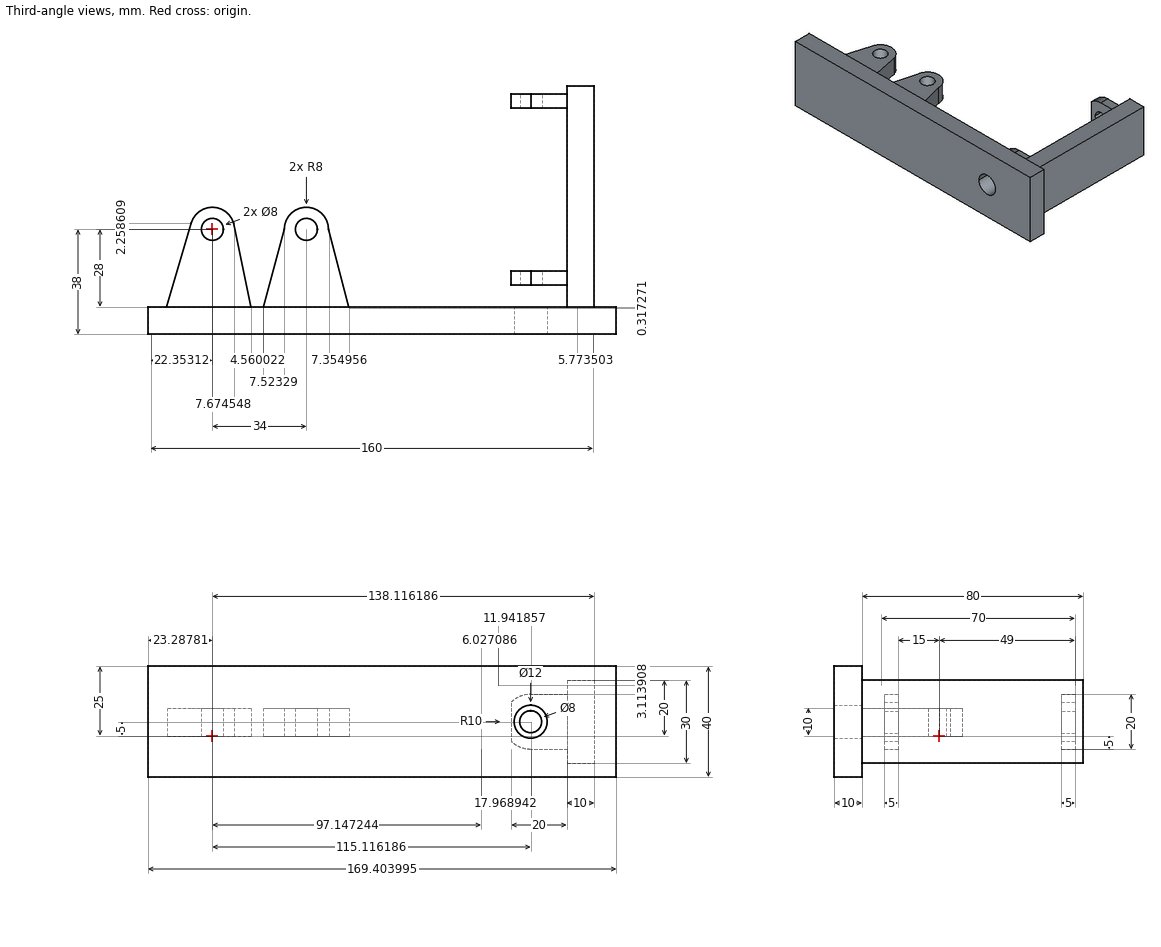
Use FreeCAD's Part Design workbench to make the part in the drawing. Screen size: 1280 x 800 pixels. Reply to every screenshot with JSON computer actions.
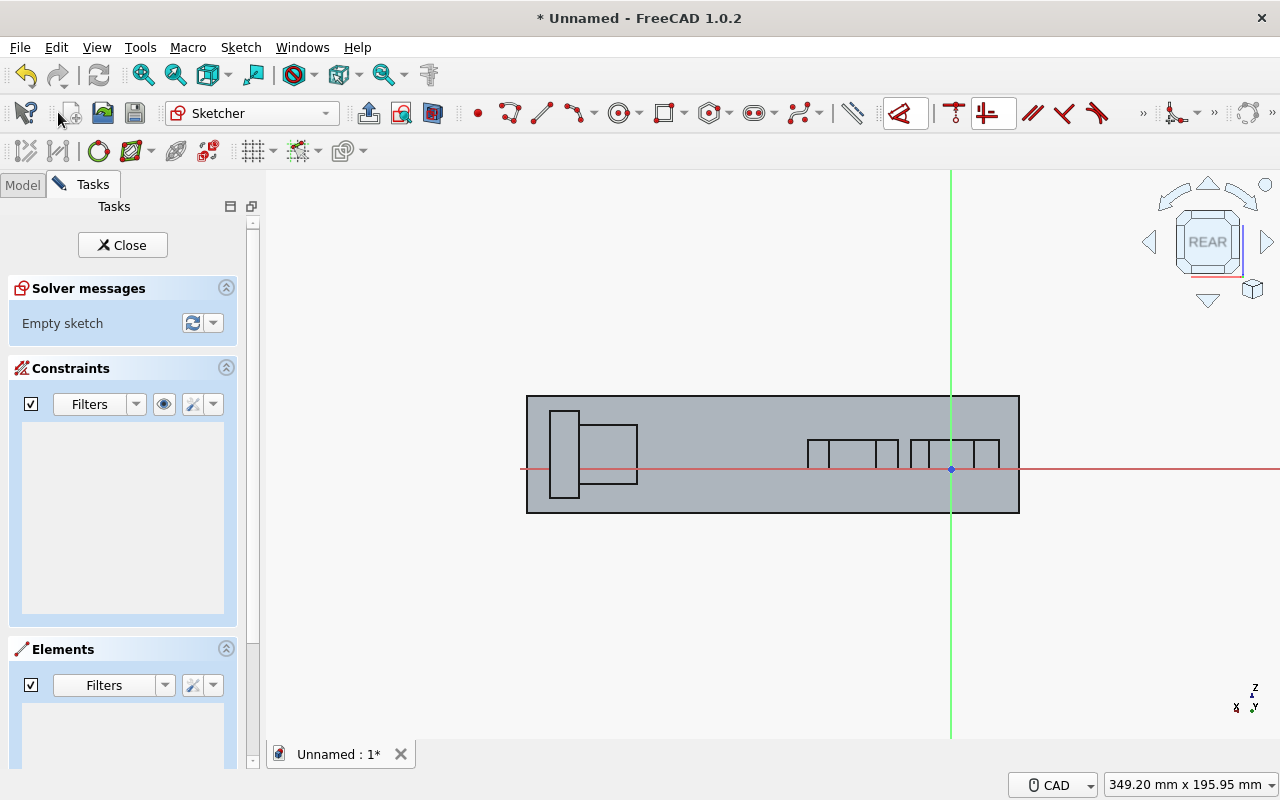
{"action": "scroll", "coordinate": [620, 449], "scroll_direction": "up", "scroll_amount": 8}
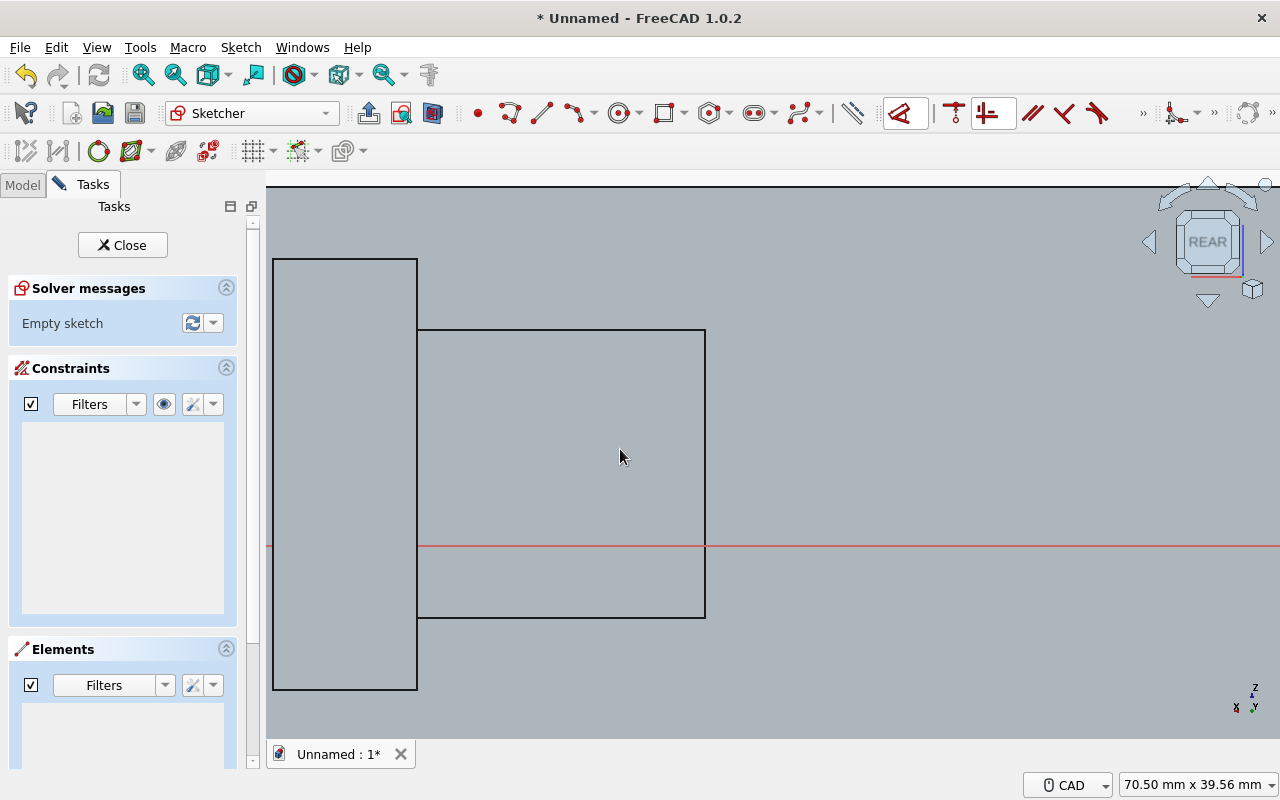
{"action": "left_click", "coordinate": [510, 114]}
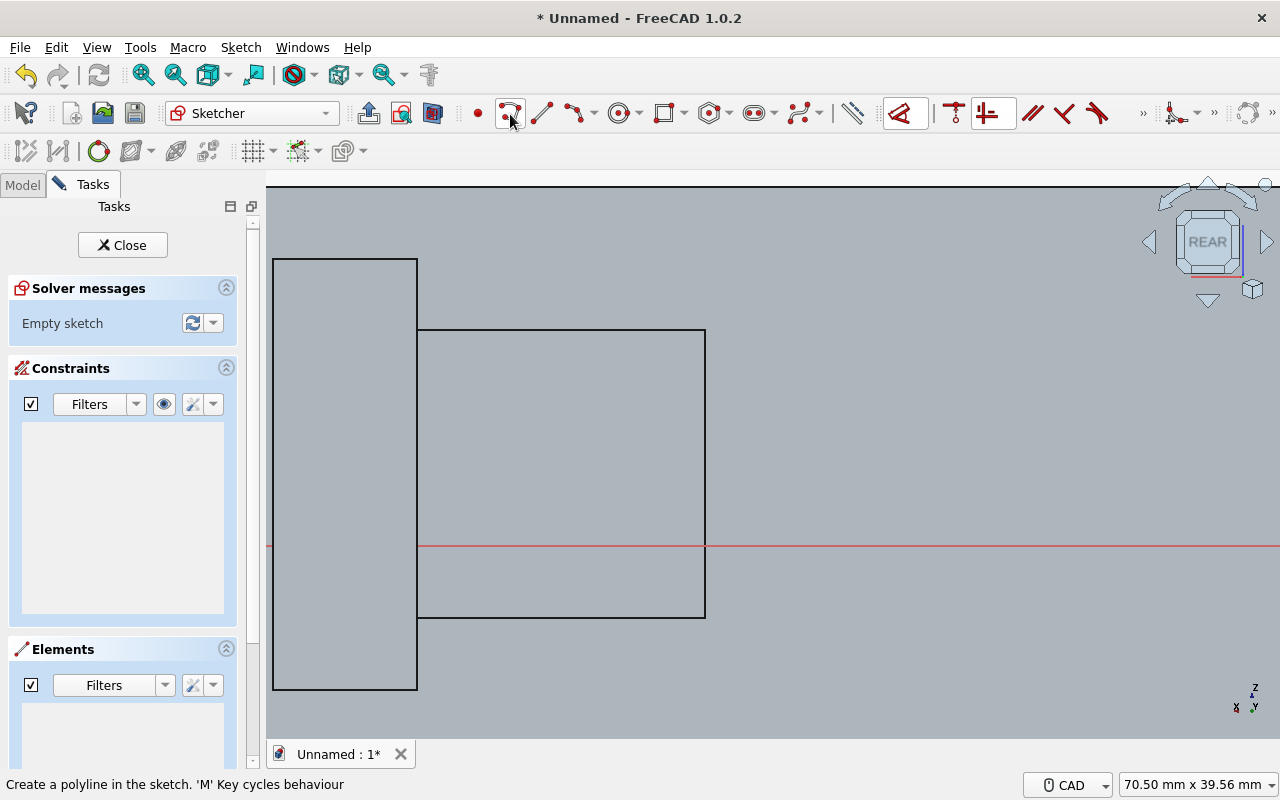
{"action": "left_click", "coordinate": [604, 618]}
{"action": "left_click", "coordinate": [863, 618]}
{"action": "left_click", "coordinate": [776, 286]}
{"action": "left_click", "coordinate": [604, 330]}
{"action": "right_click", "coordinate": [604, 330]}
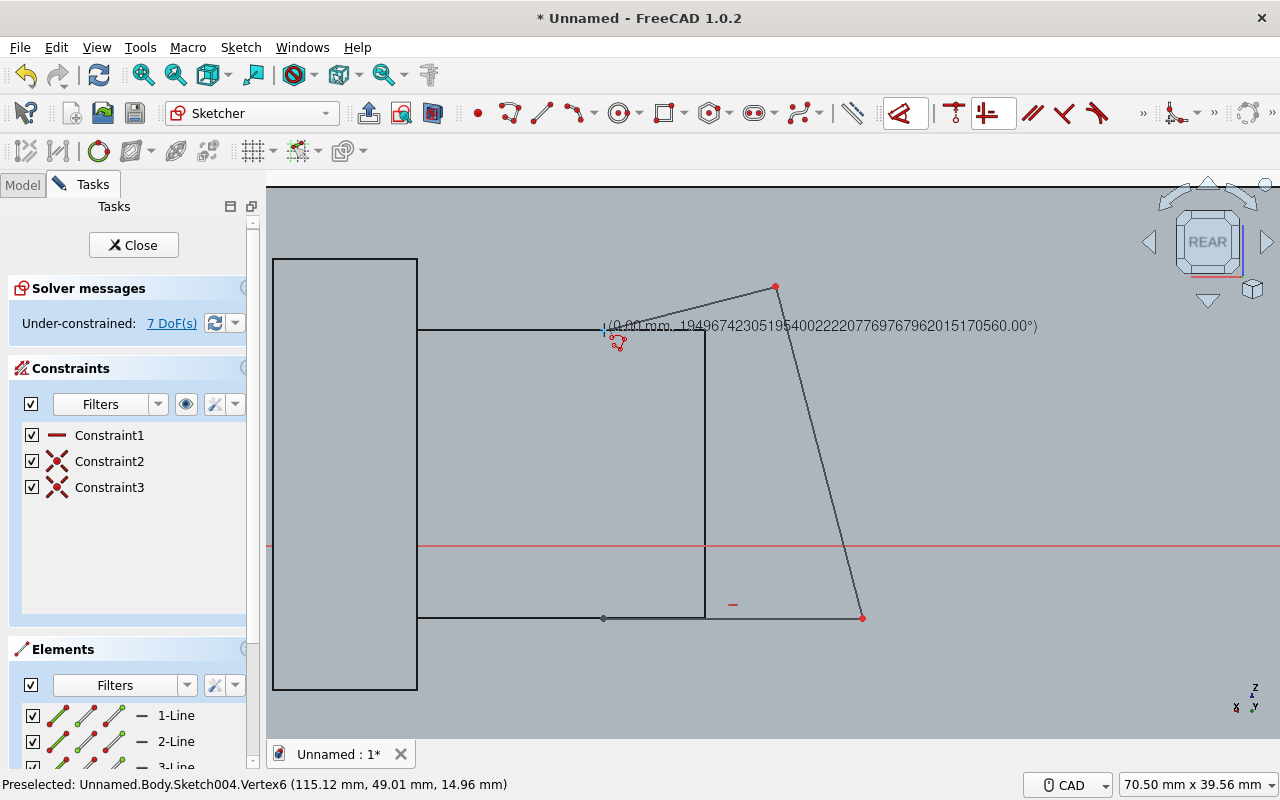
{"action": "left_click", "coordinate": [574, 114]}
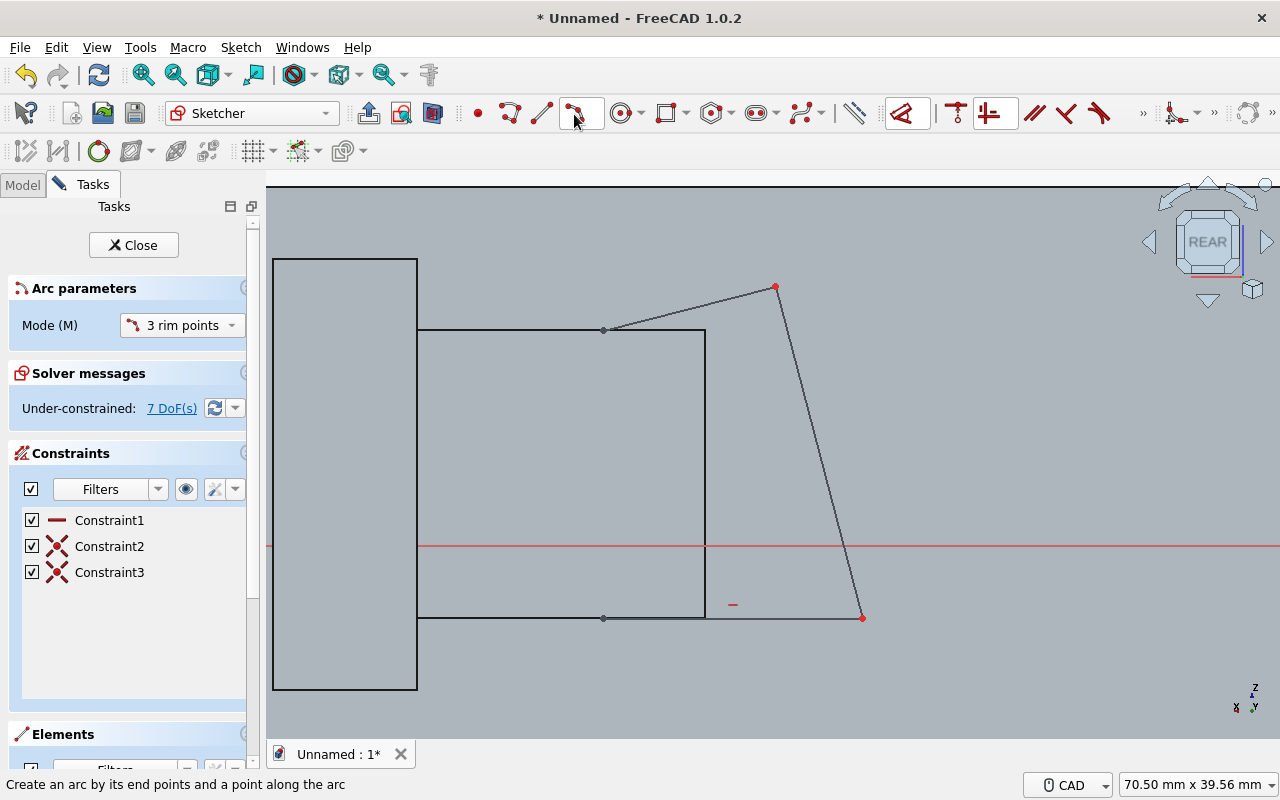
{"action": "left_click", "coordinate": [604, 331]}
{"action": "left_click", "coordinate": [604, 619]}
{"action": "left_click", "coordinate": [748, 474]}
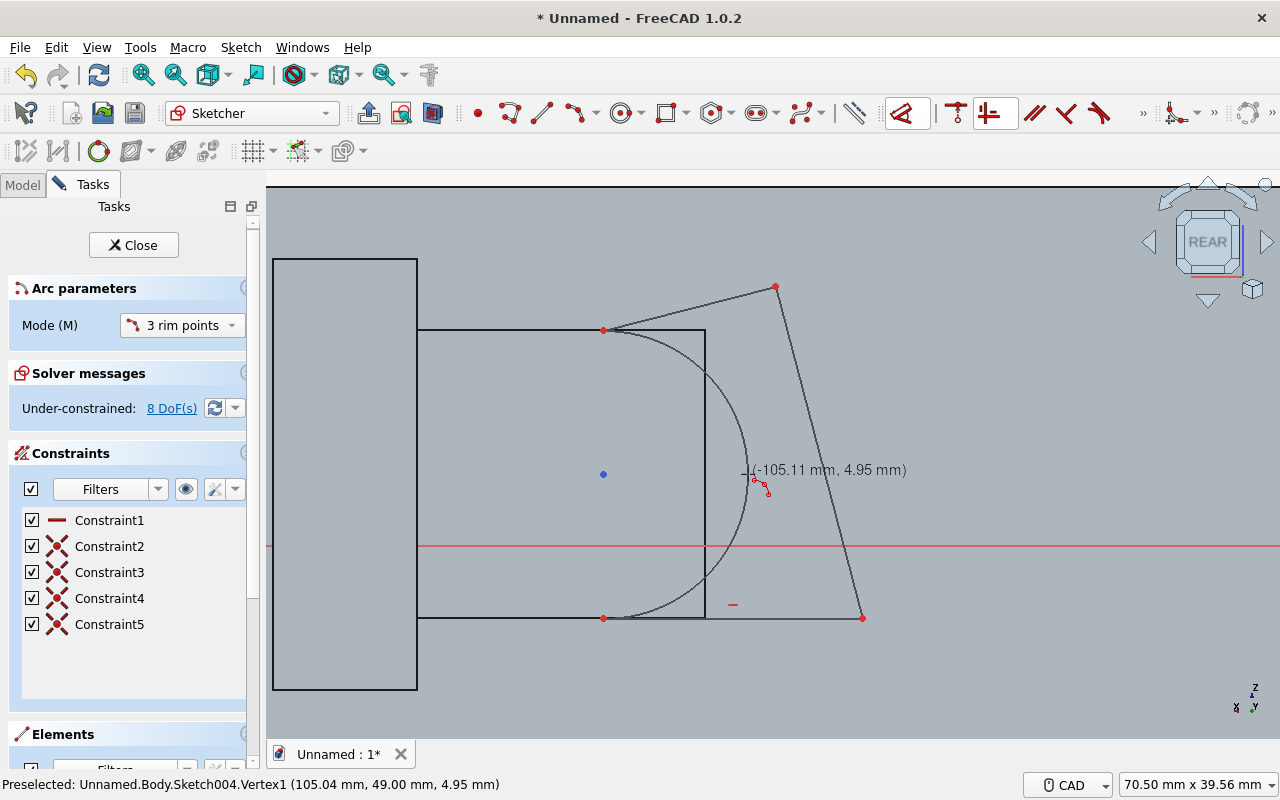
{"action": "left_click", "coordinate": [622, 114]}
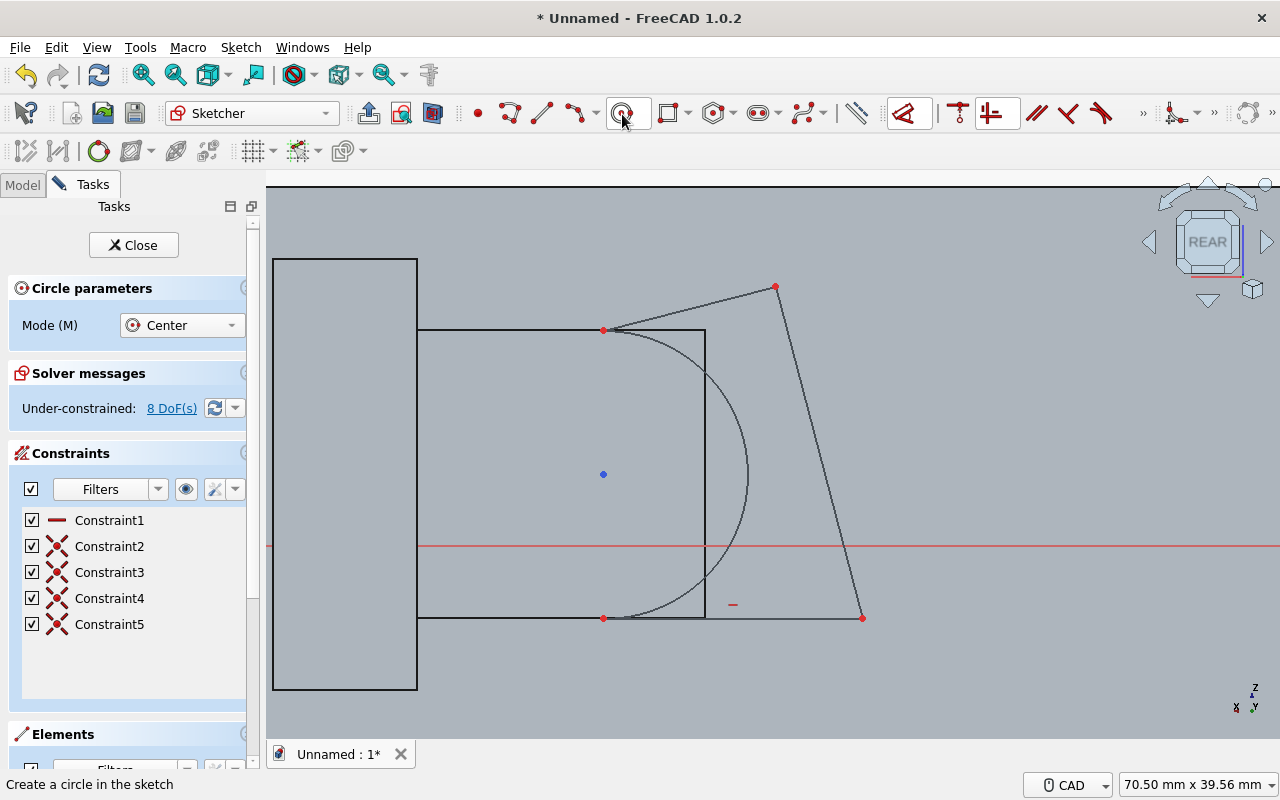
{"action": "left_click", "coordinate": [604, 474]}
{"action": "mouse_move", "coordinate": [645, 434]}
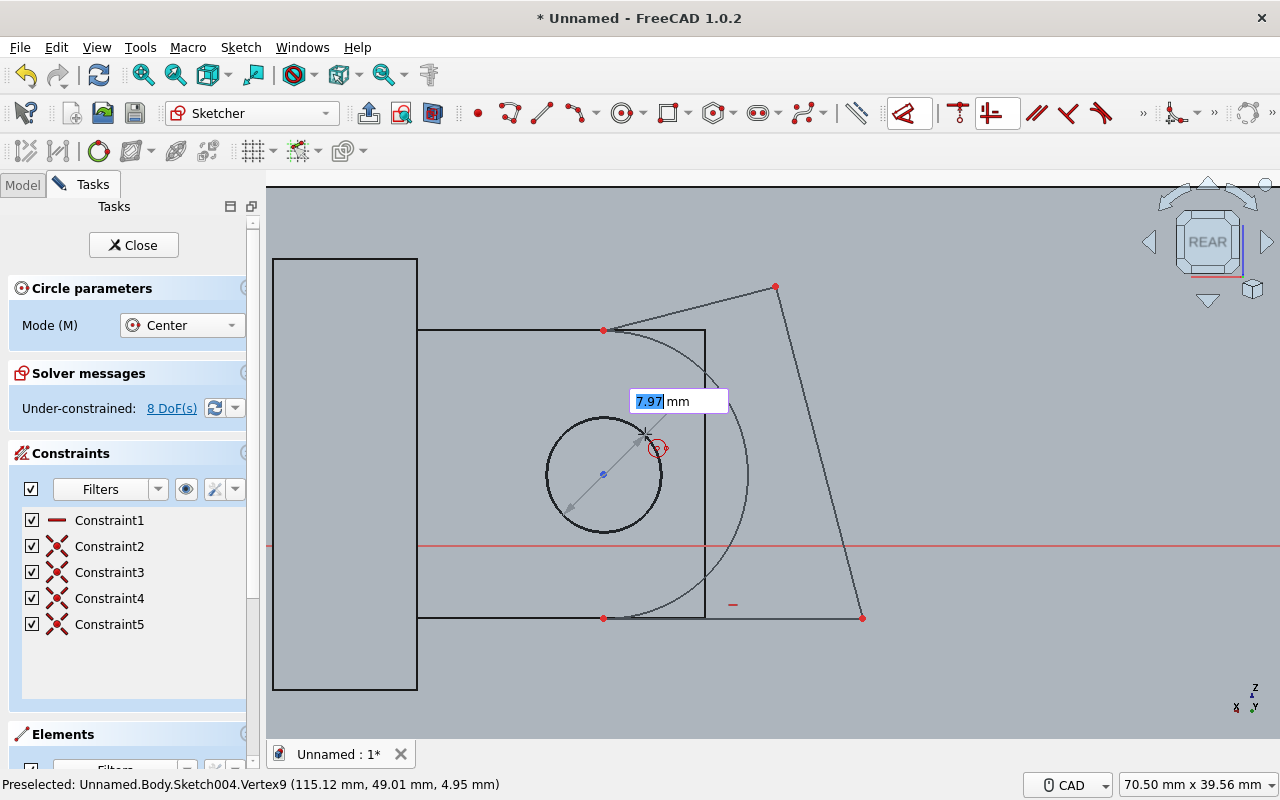
{"action": "type", "text": "8"}
{"action": "key", "text": "Return"}
{"action": "key", "text": "Escape"}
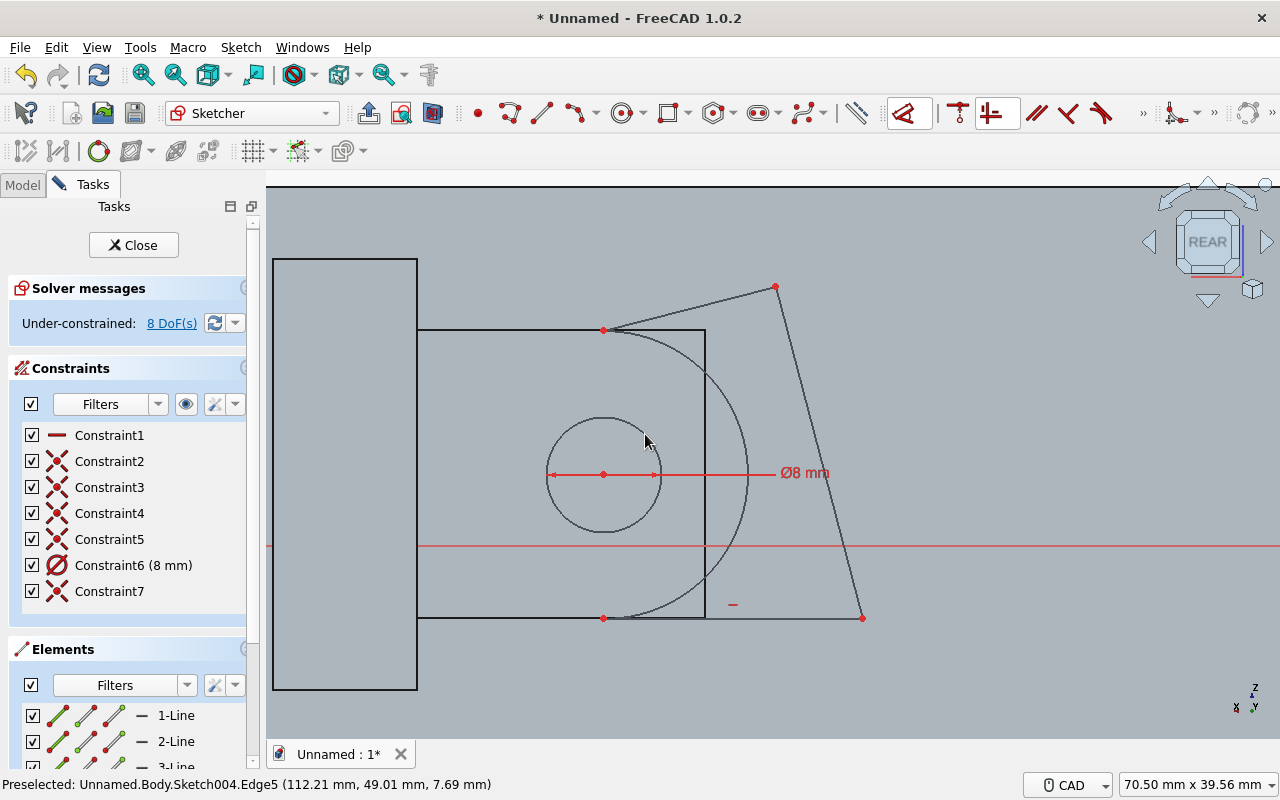
{"action": "left_click", "coordinate": [682, 619]}